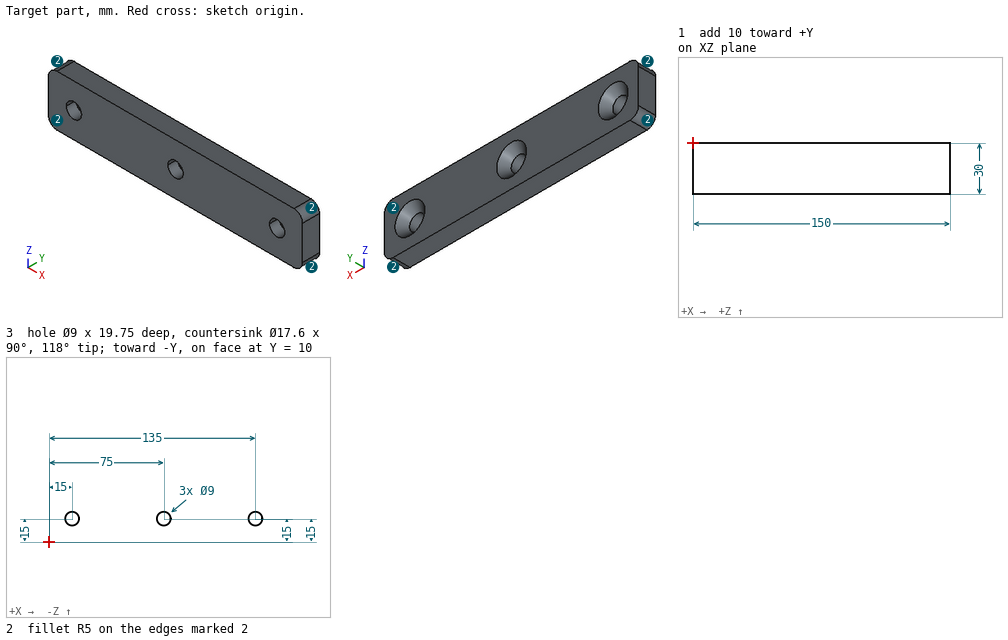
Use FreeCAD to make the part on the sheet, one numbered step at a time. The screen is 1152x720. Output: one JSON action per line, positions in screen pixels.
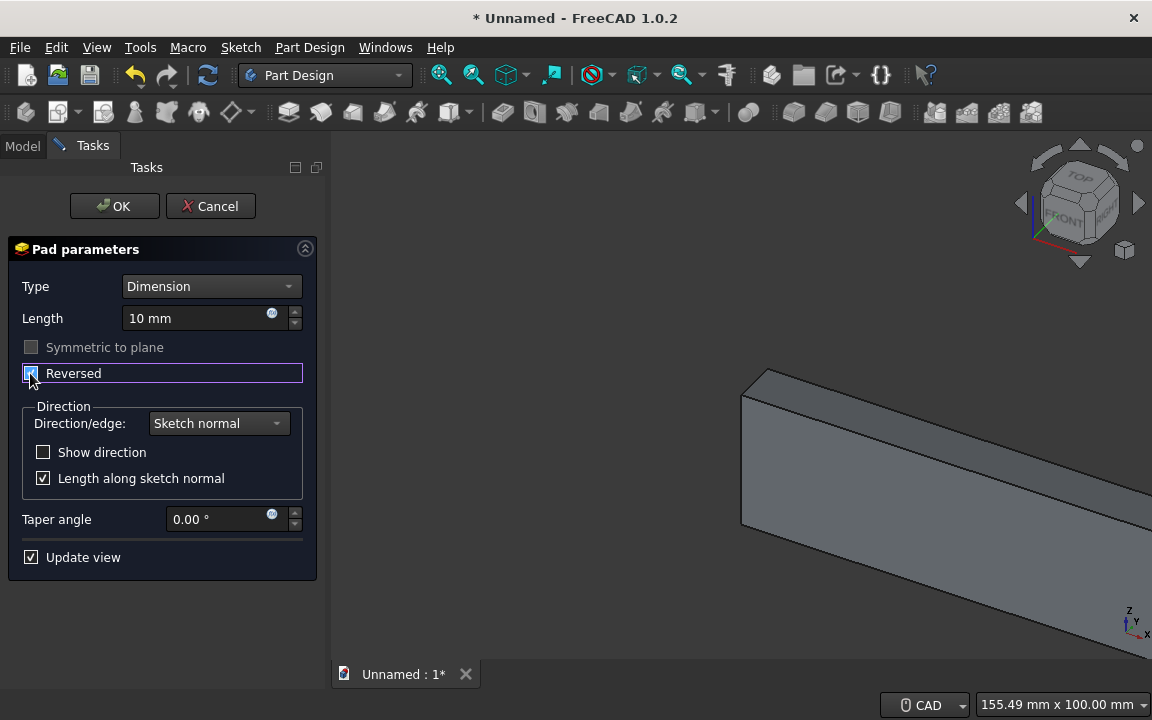
{"action": "left_click", "coordinate": [115, 206]}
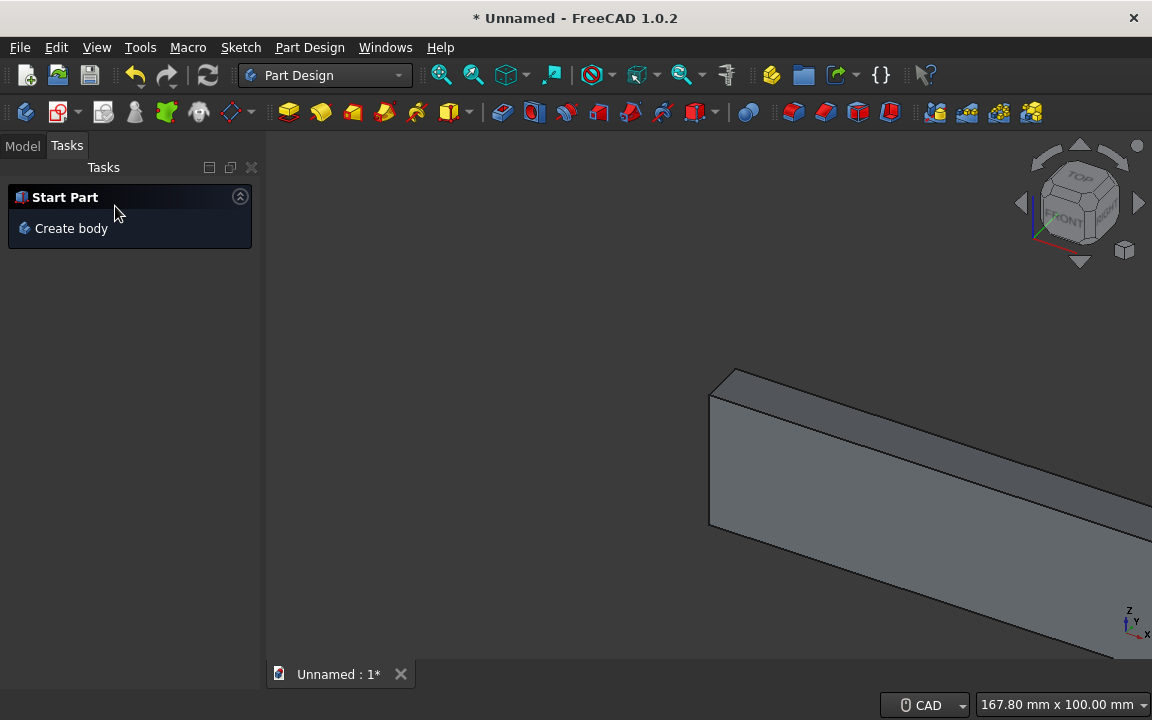
{"action": "left_click", "coordinate": [442, 76]}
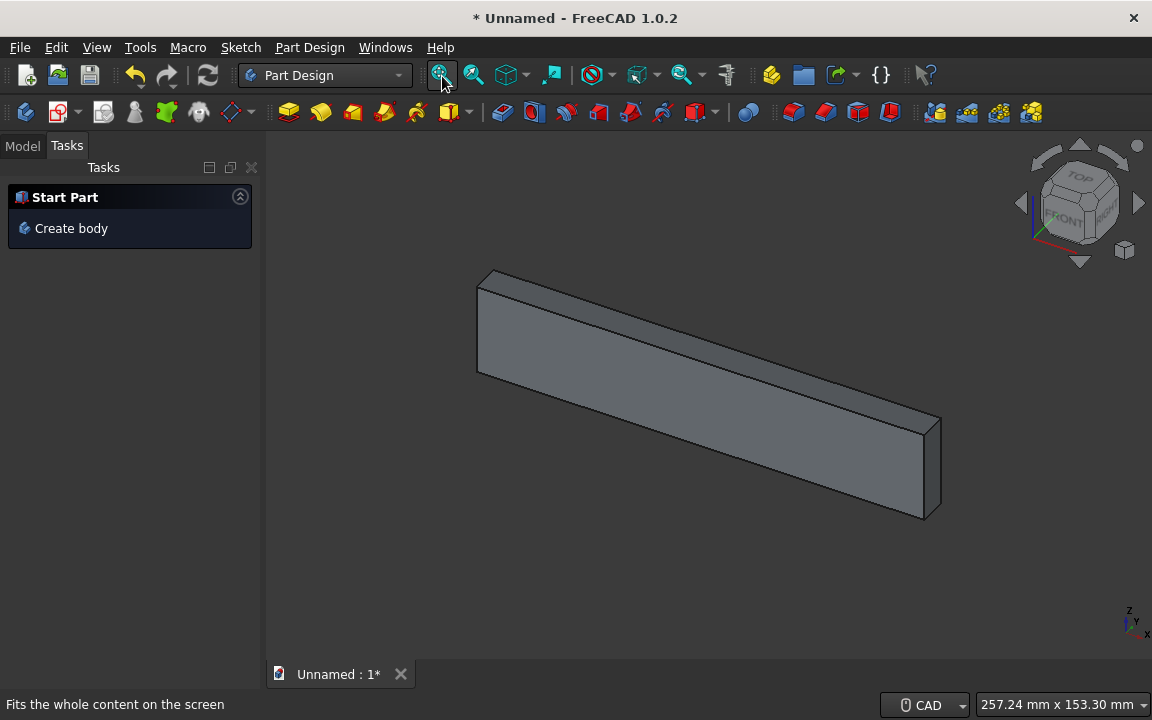
{"action": "left_click", "coordinate": [933, 426]}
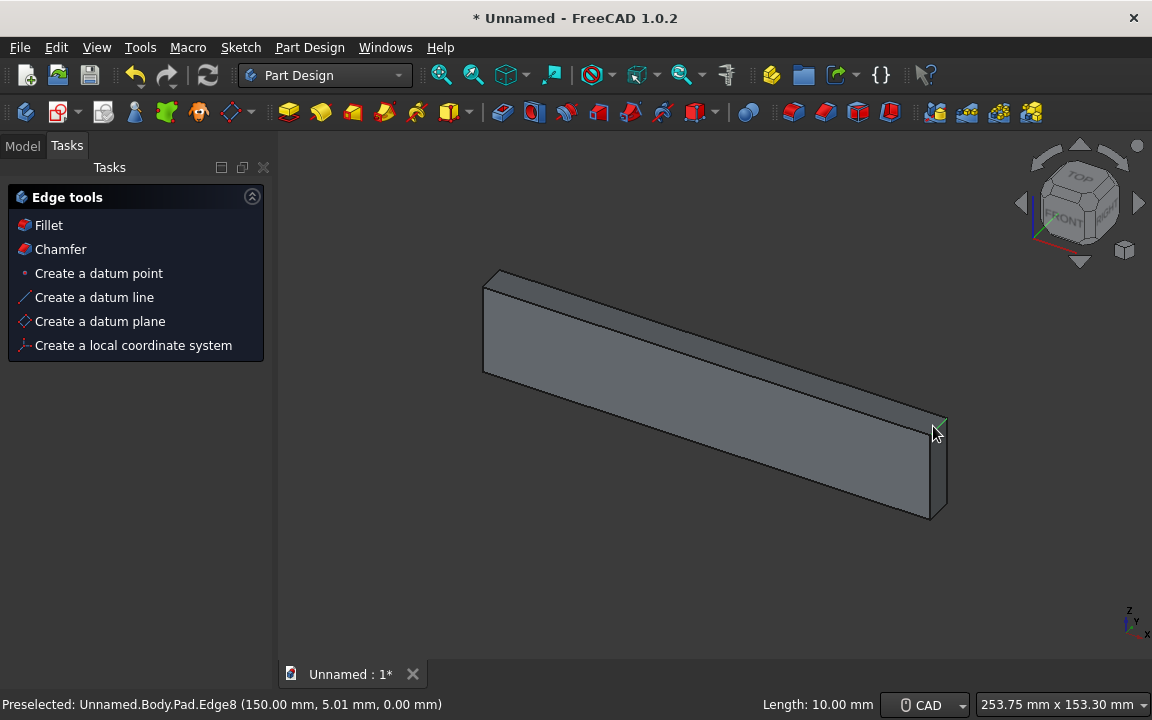
{"action": "key", "text": "0"}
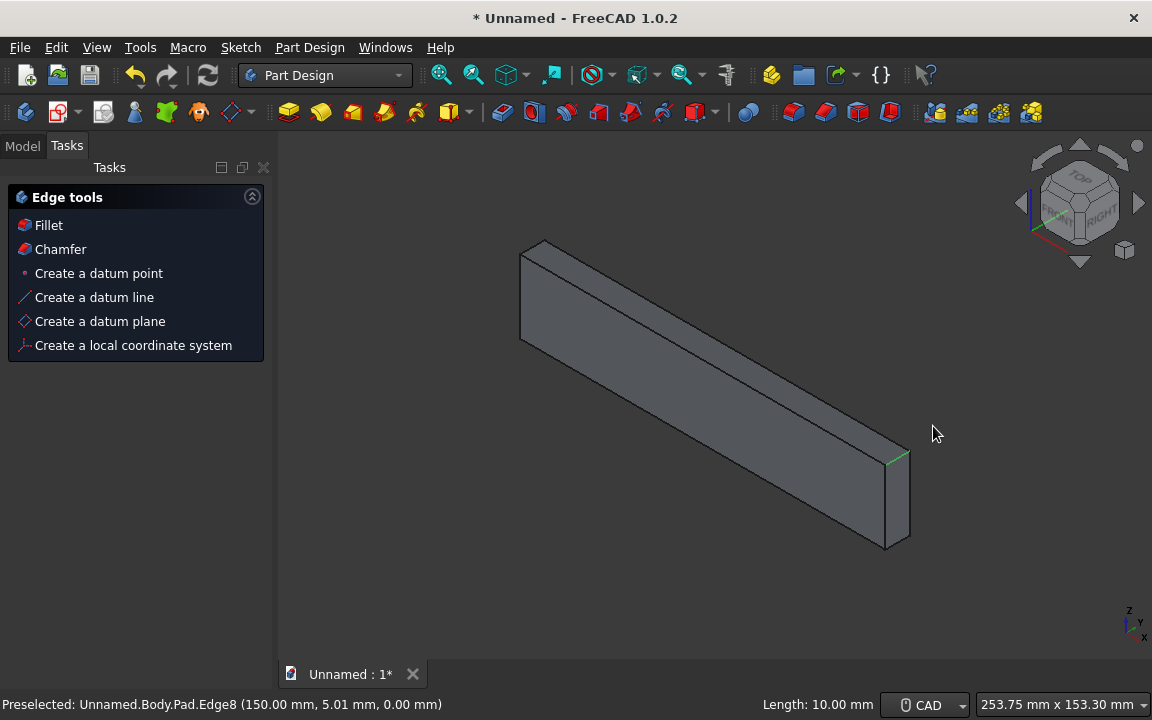
{"action": "key", "text": "2"}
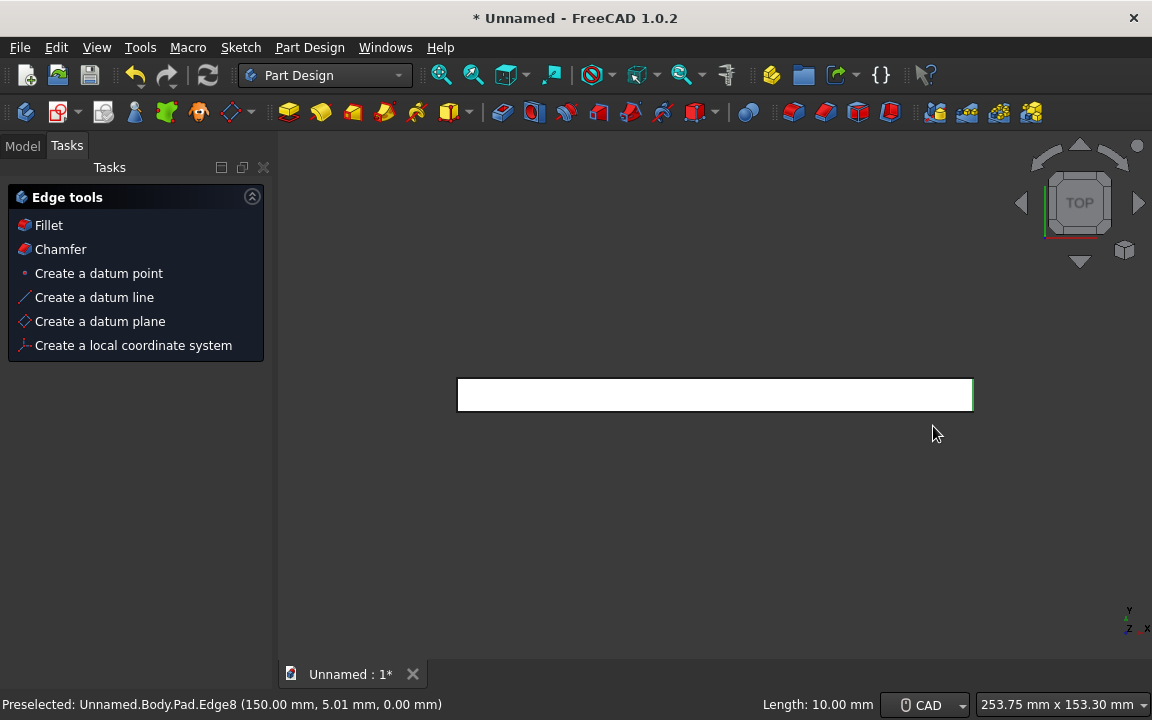
{"action": "left_click", "coordinate": [457, 394], "text": "ctrl"}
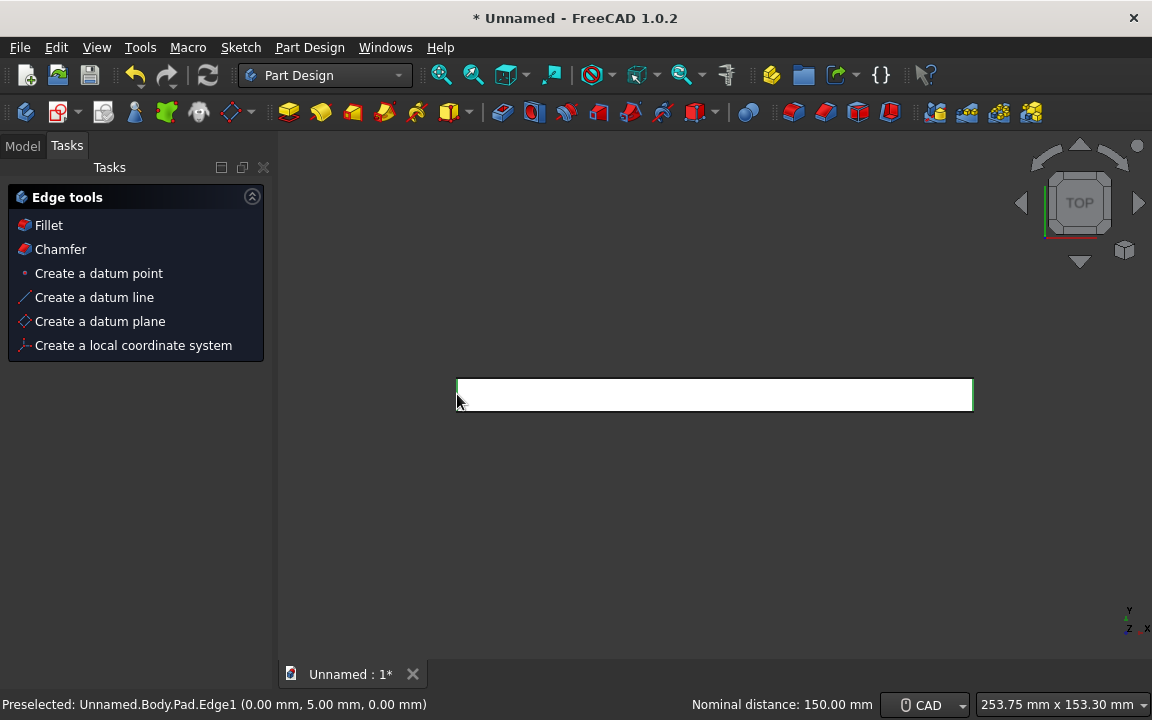
{"action": "key", "text": "1"}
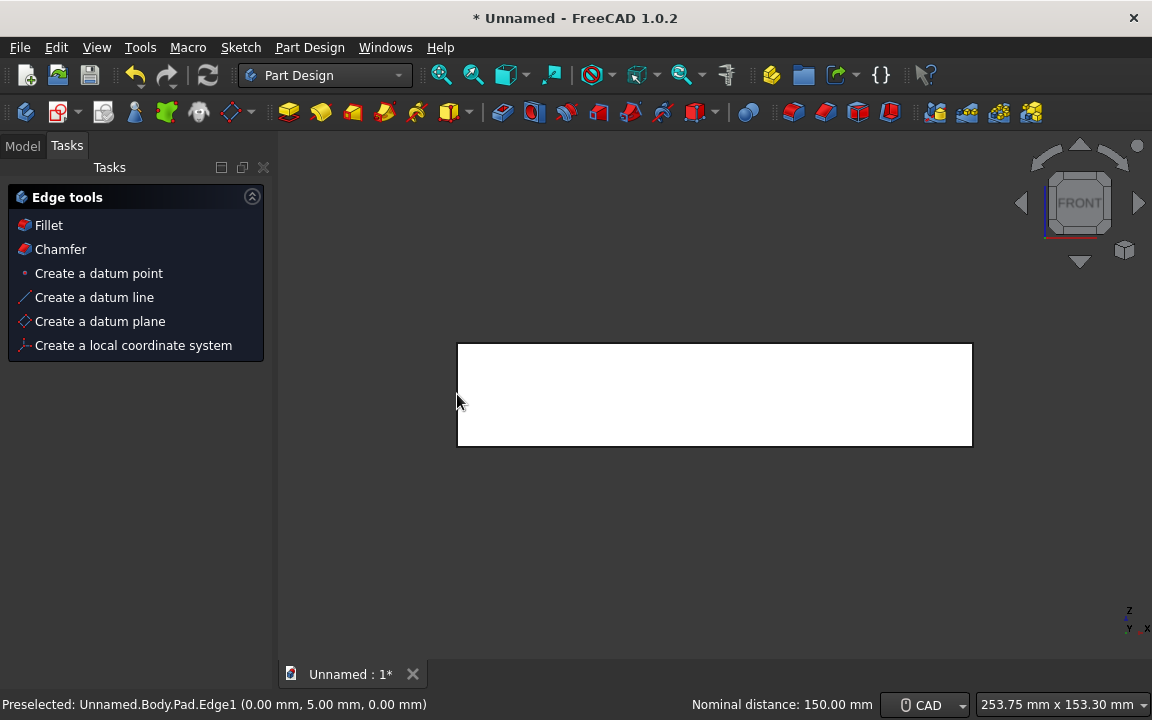
{"action": "key", "text": "3"}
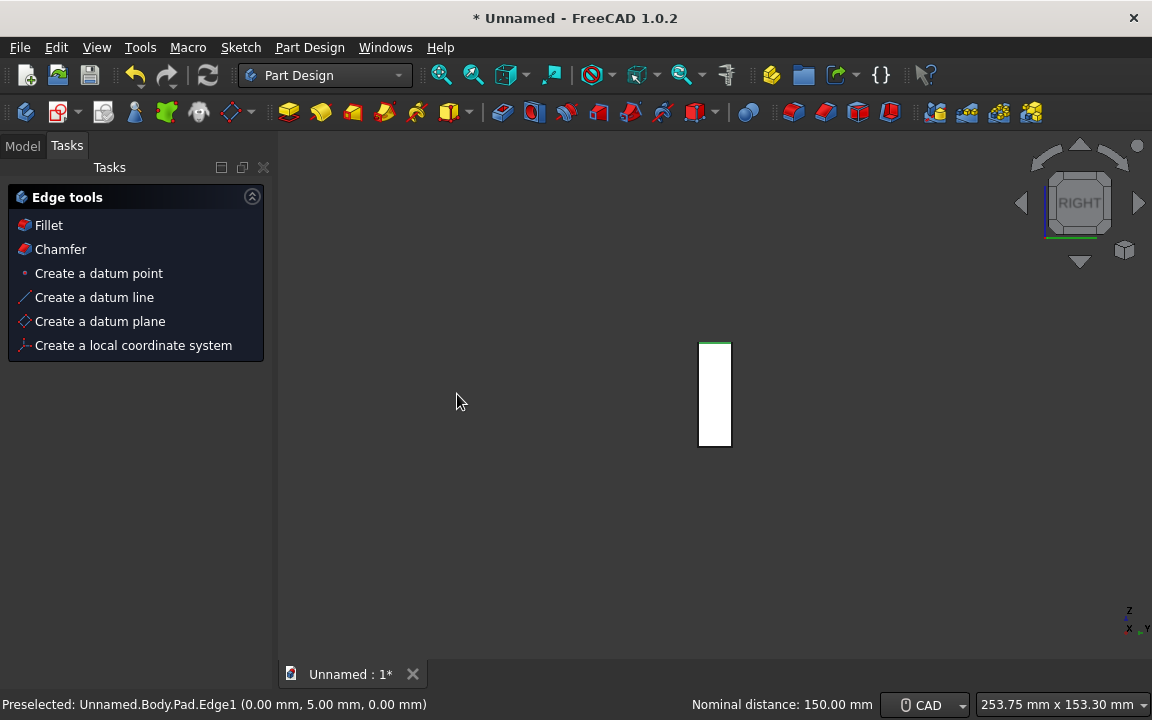
{"action": "left_click", "coordinate": [442, 76]}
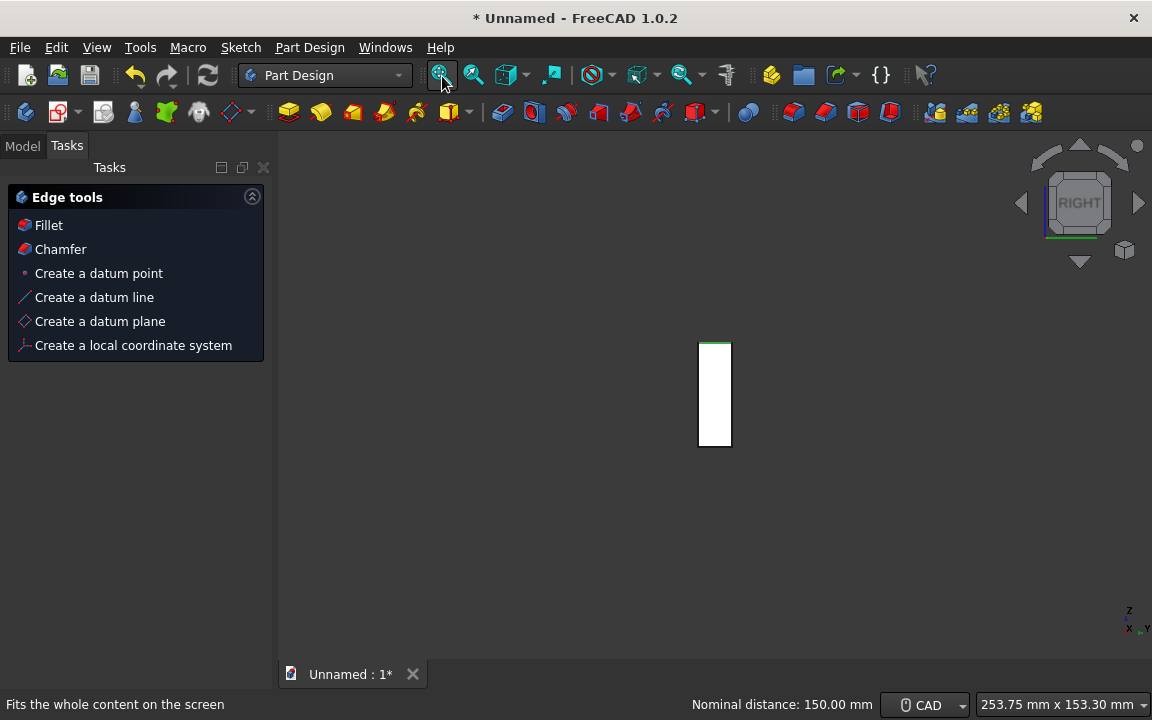
{"action": "left_click", "coordinate": [715, 446], "text": "ctrl"}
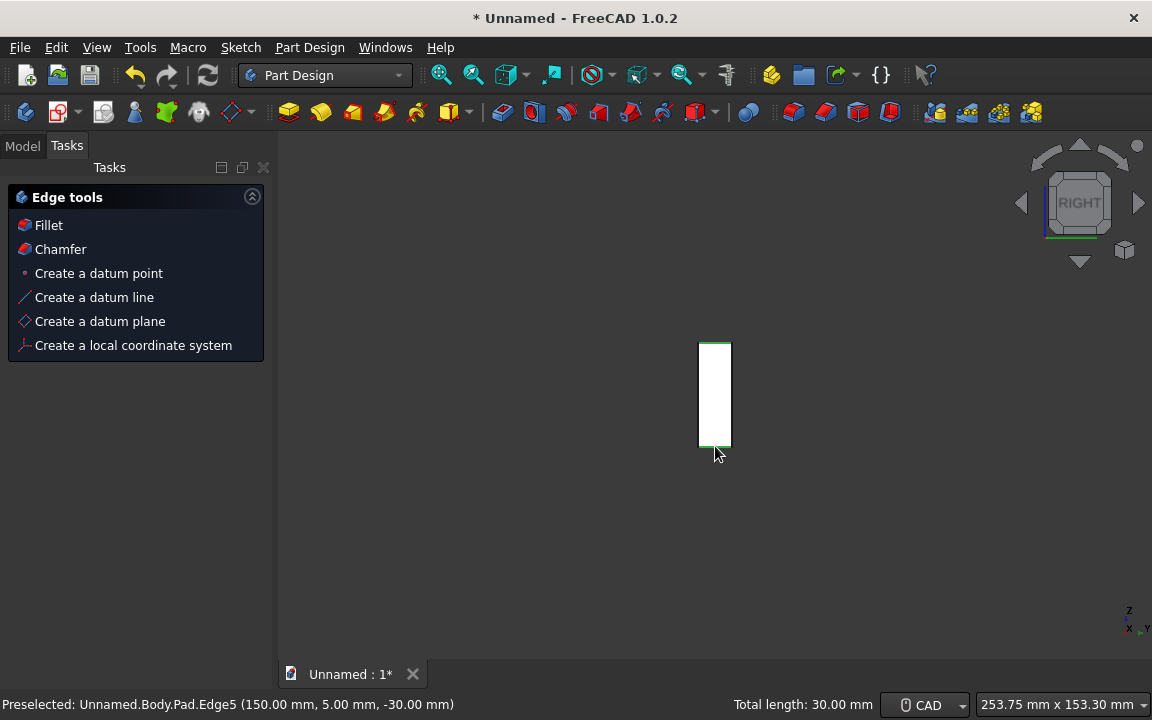
{"action": "key", "text": "5"}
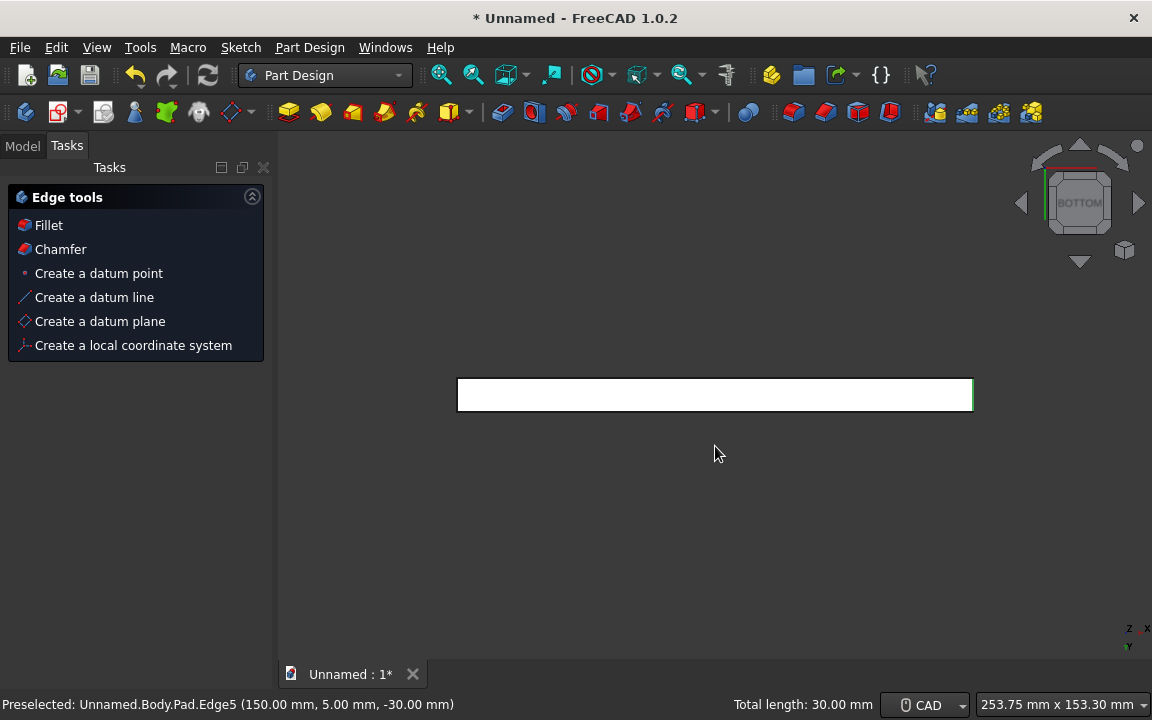
{"action": "left_click", "coordinate": [457, 394], "text": "ctrl"}